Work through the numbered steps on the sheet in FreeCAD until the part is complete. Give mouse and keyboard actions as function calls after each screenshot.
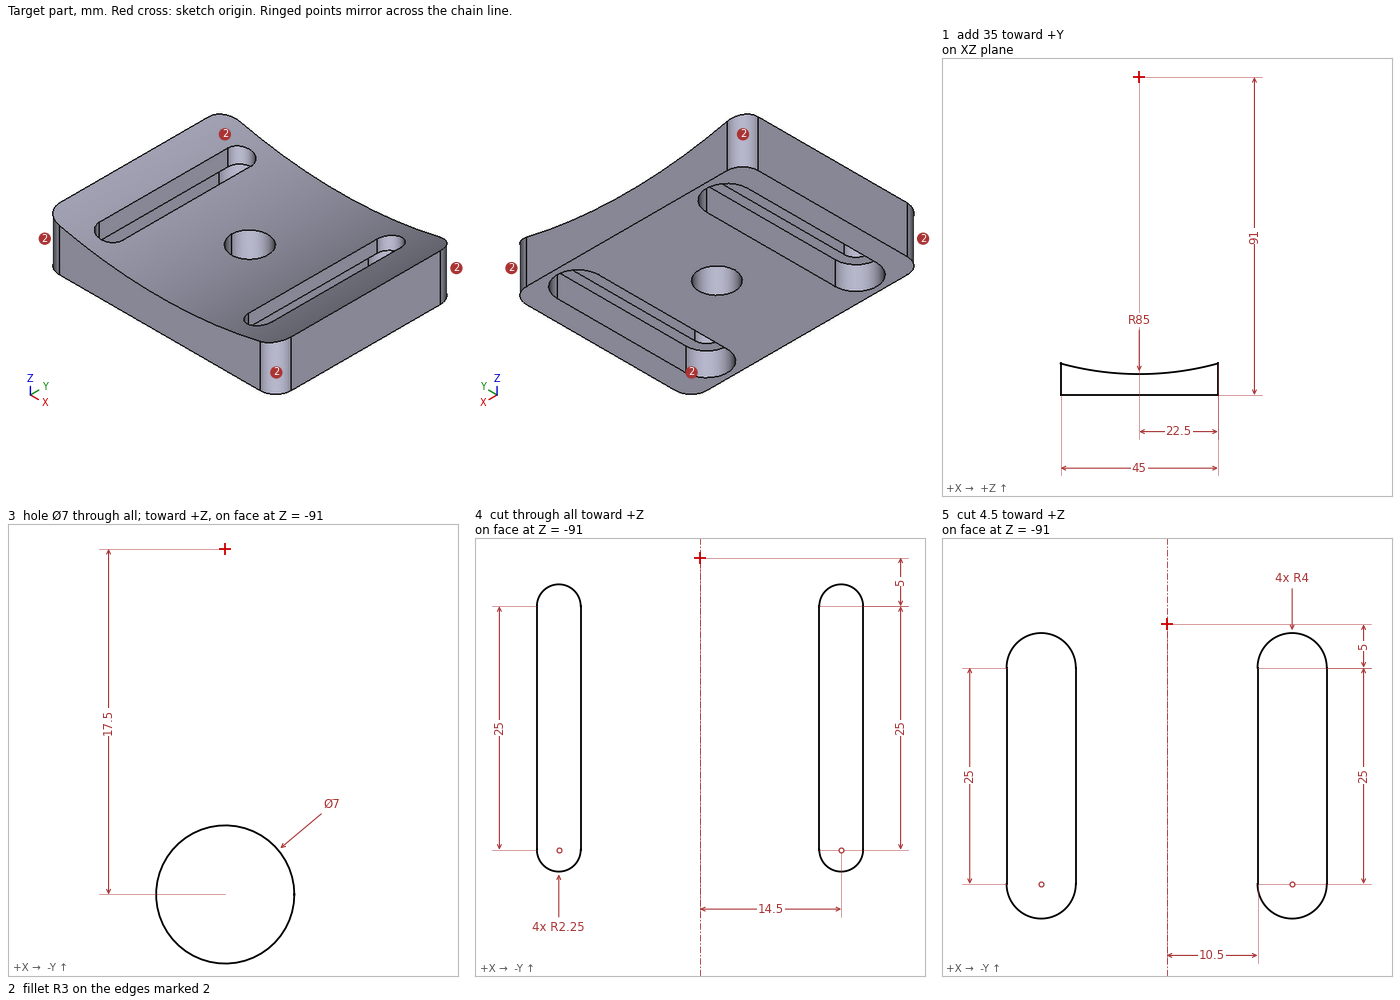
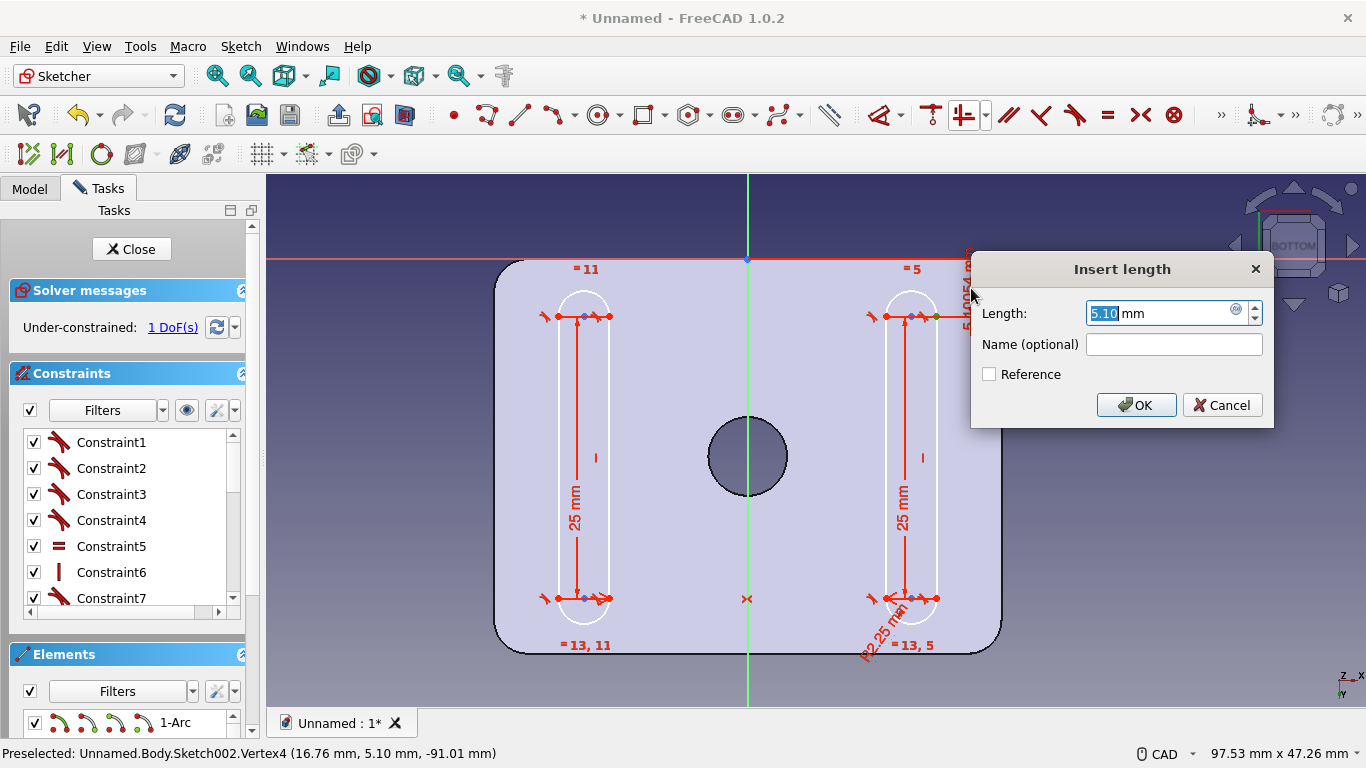
text(5)
key(Return)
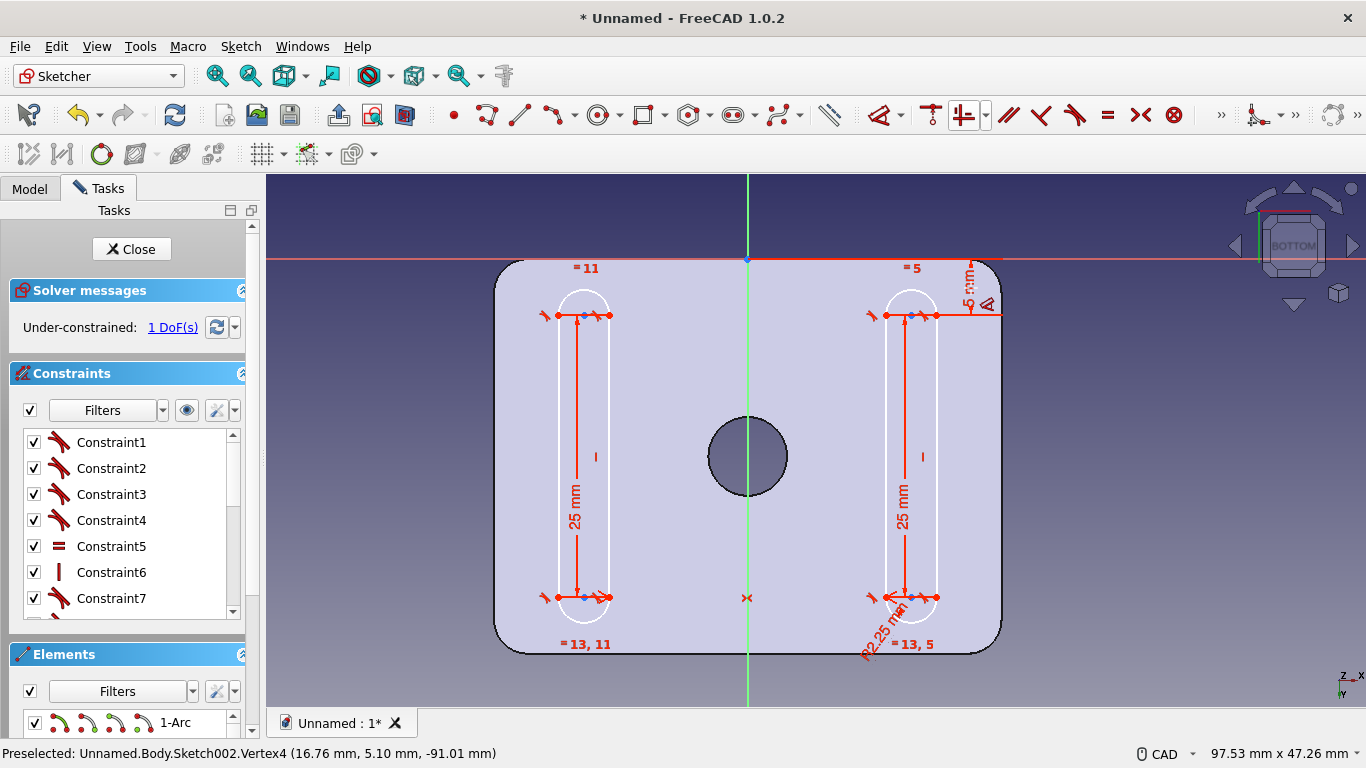
click(911, 597)
click(830, 225)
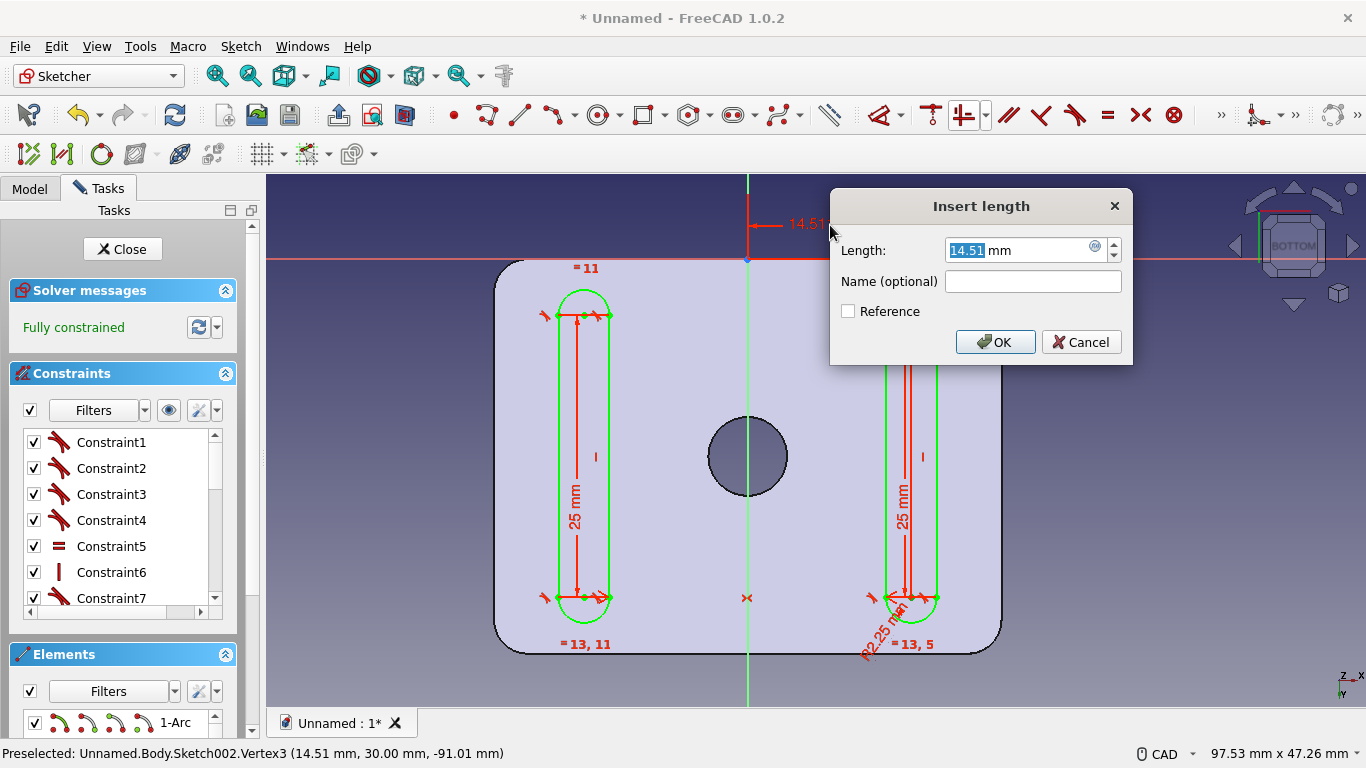
text(14.5)
key(Return)
key(Escape)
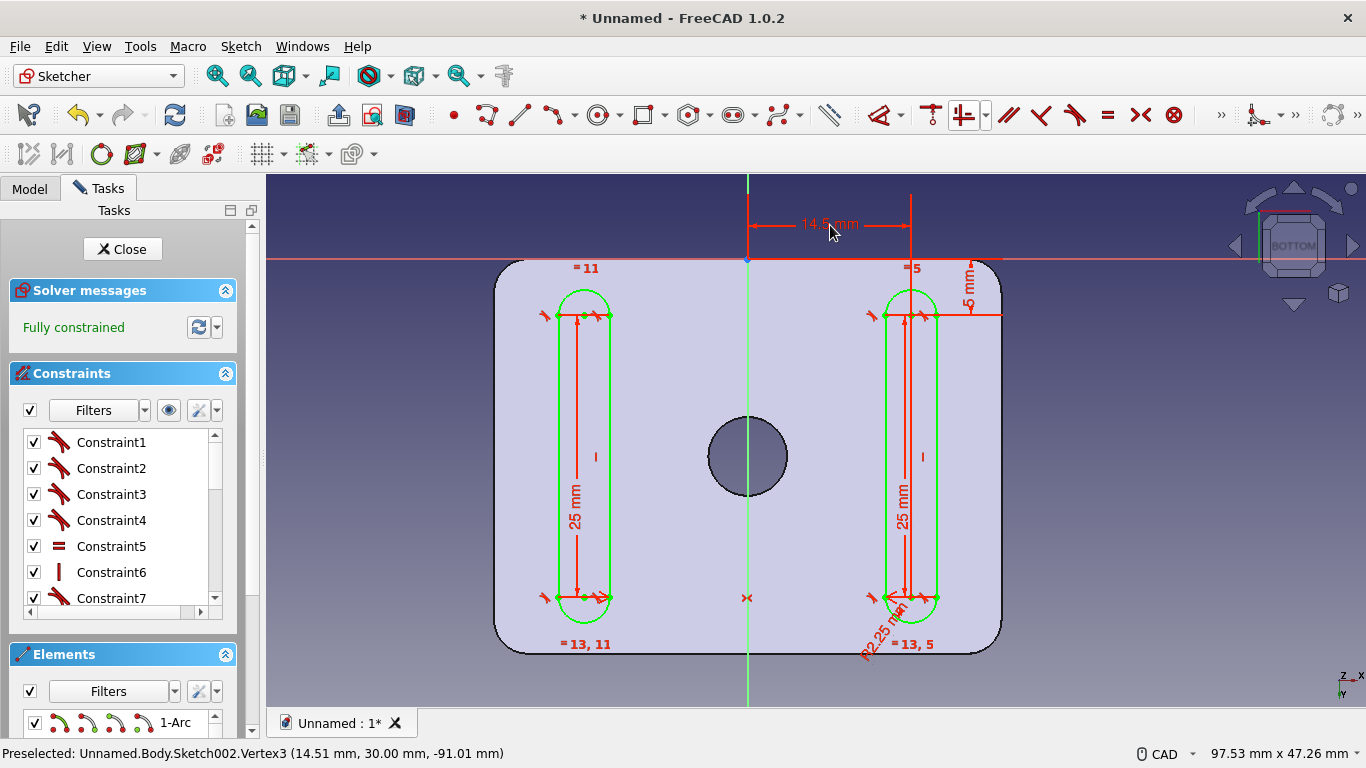
click(123, 249)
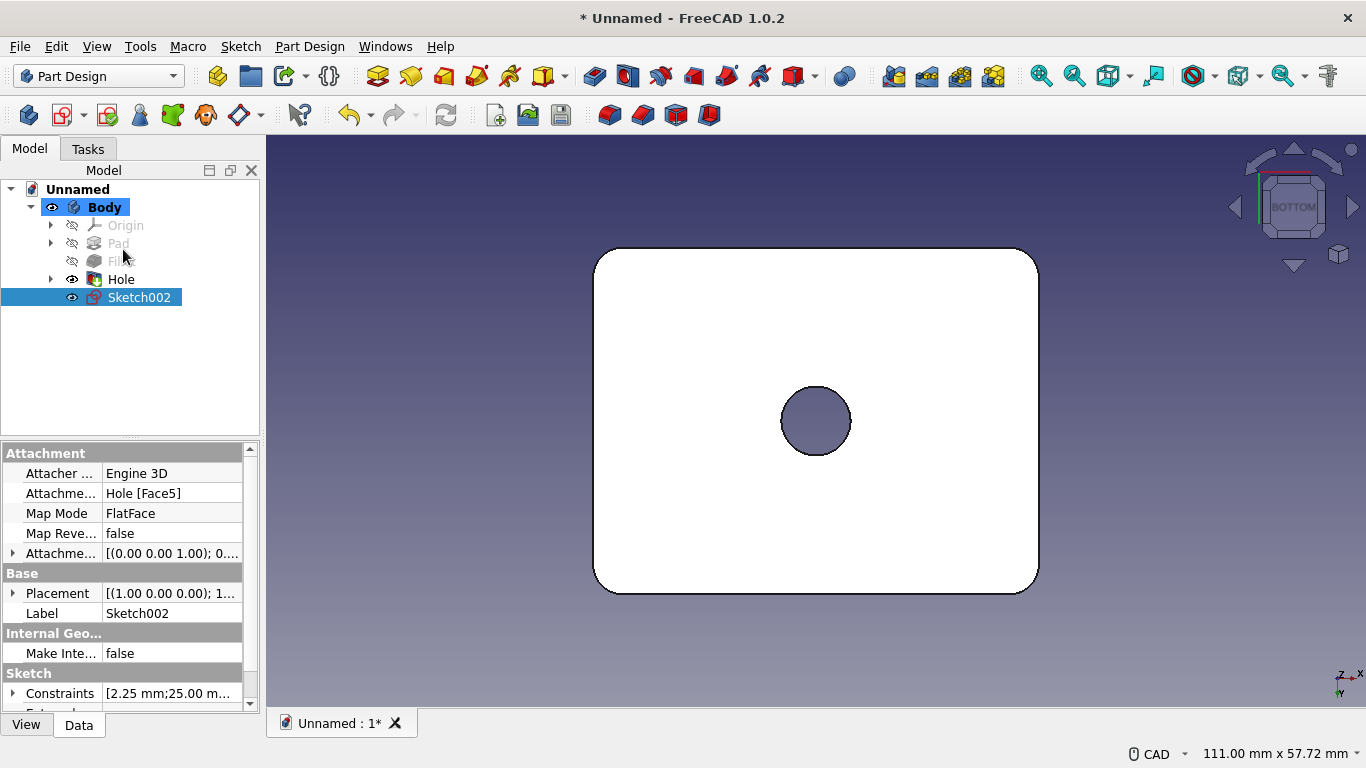
click(595, 76)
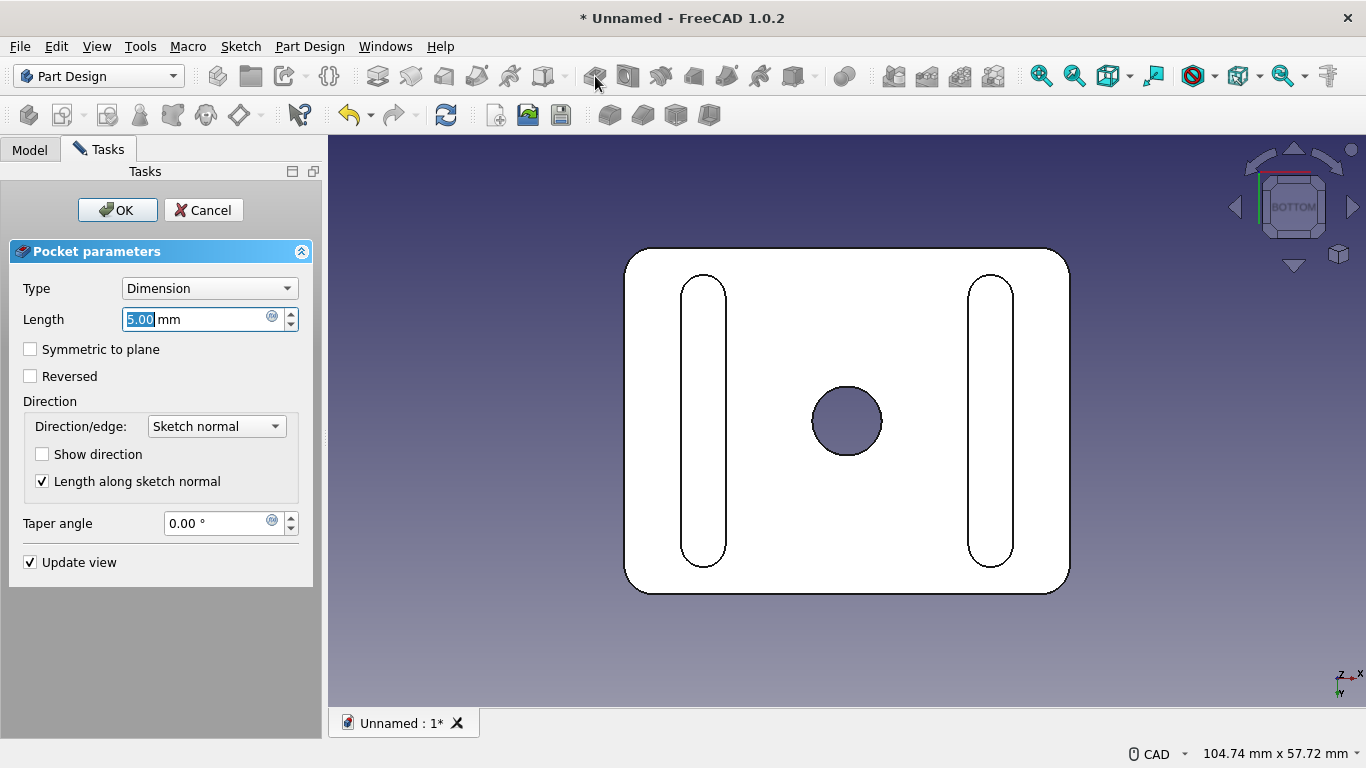
click(210, 288)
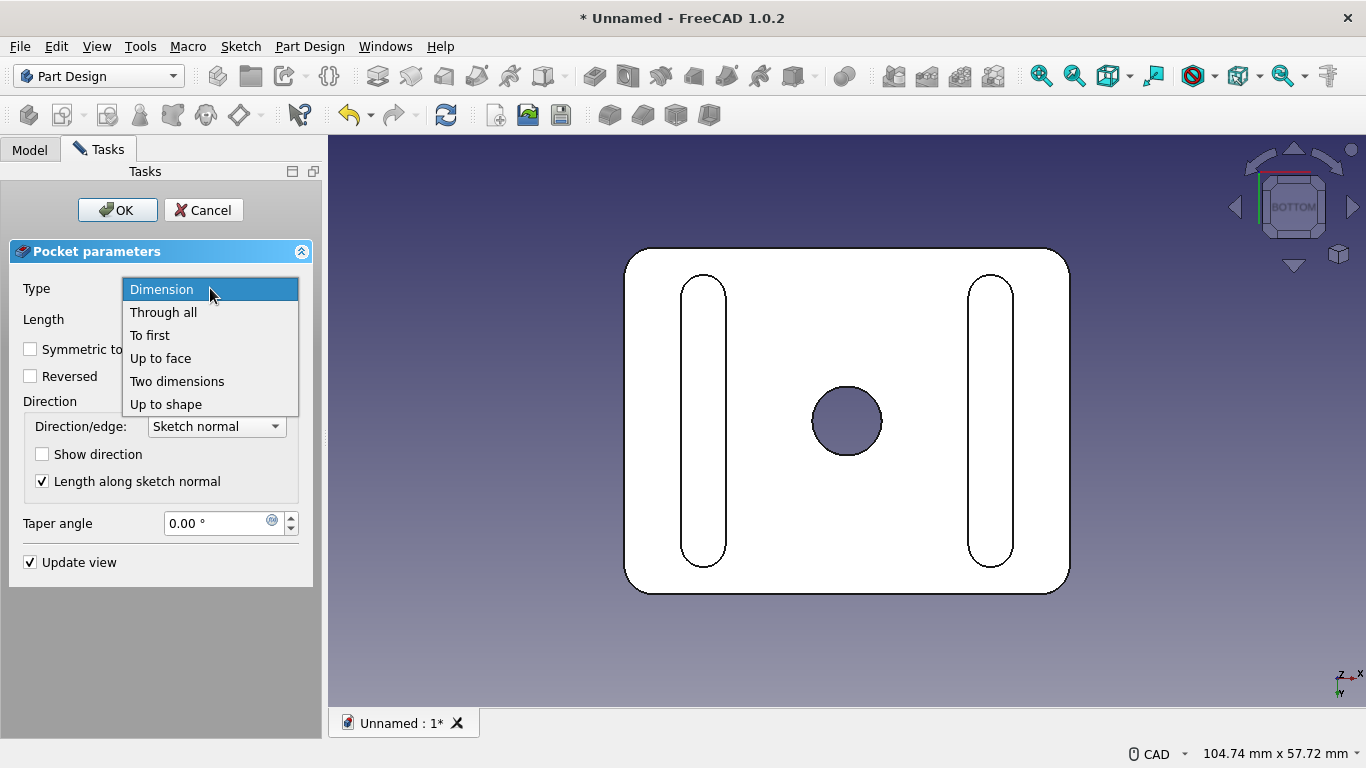
click(208, 312)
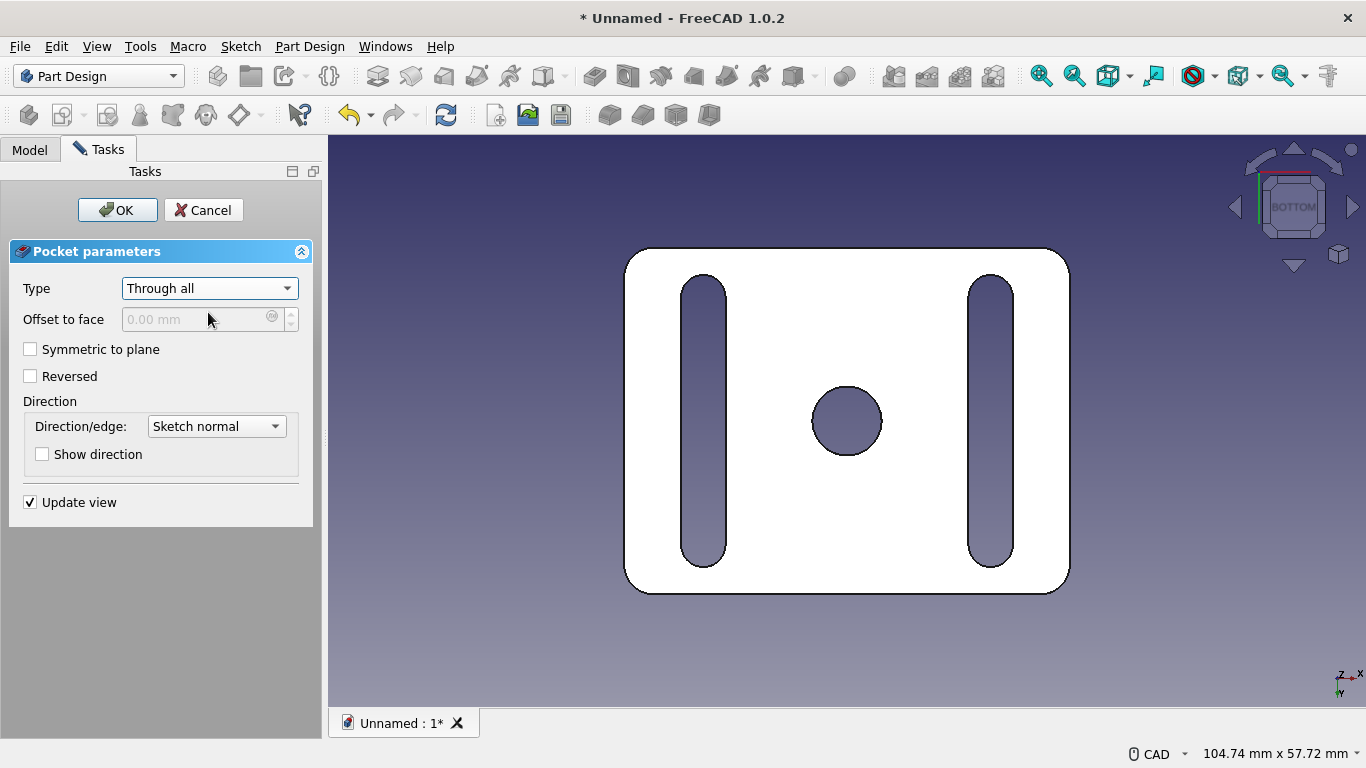
click(118, 210)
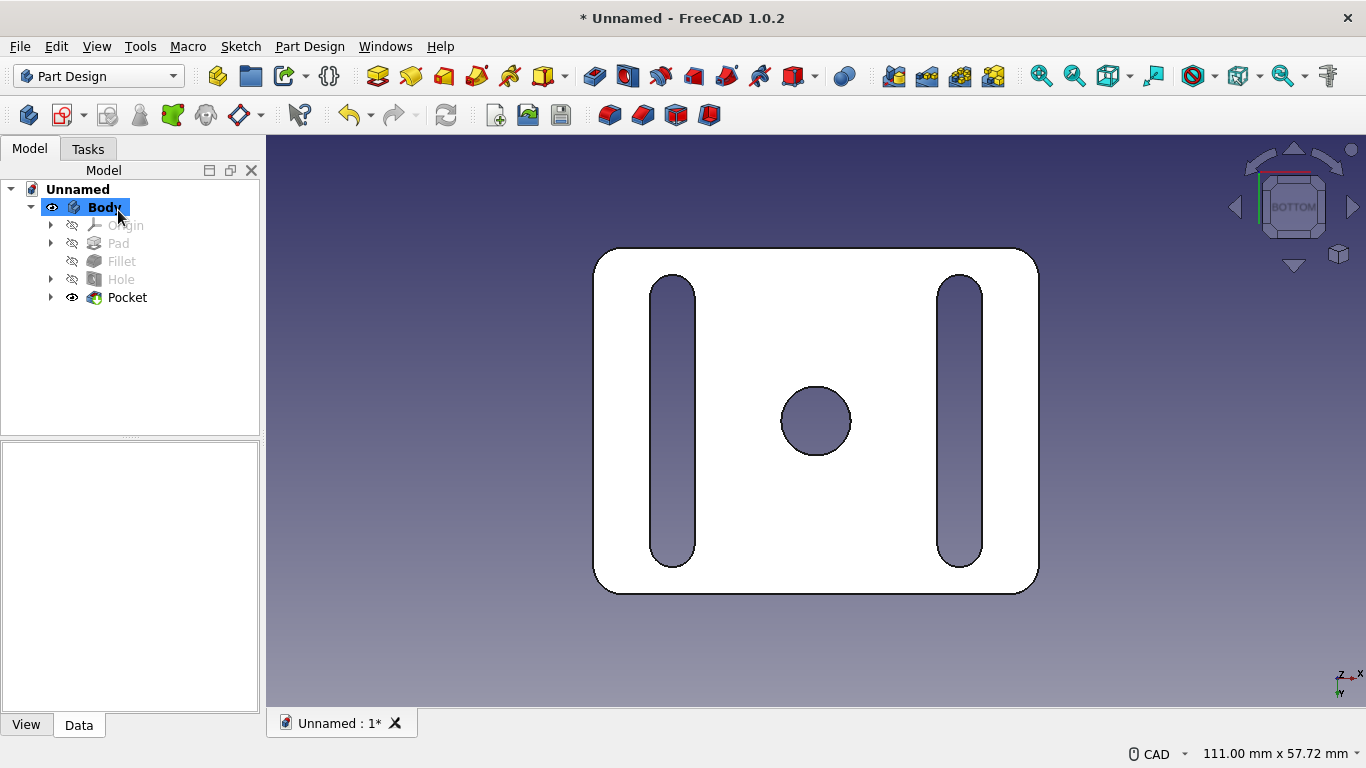
click(816, 519)